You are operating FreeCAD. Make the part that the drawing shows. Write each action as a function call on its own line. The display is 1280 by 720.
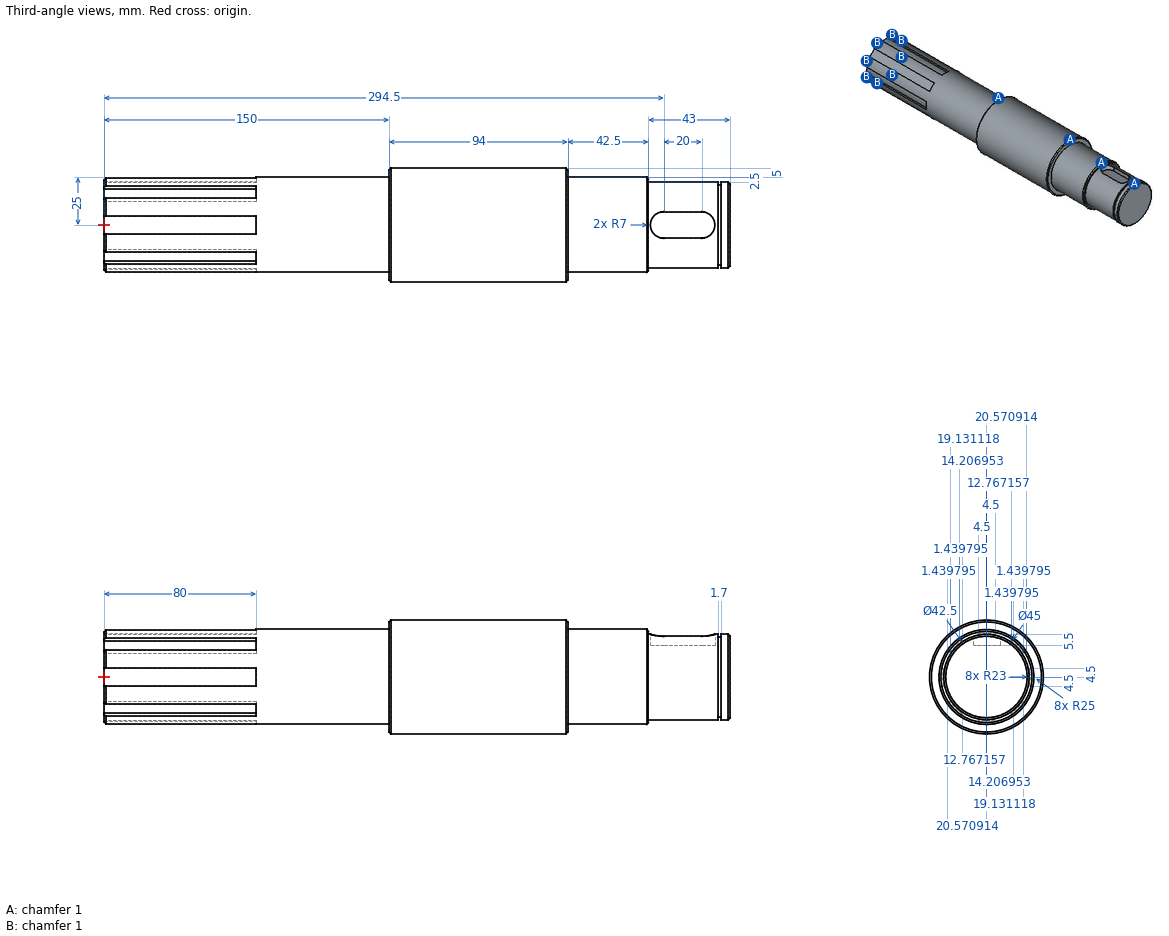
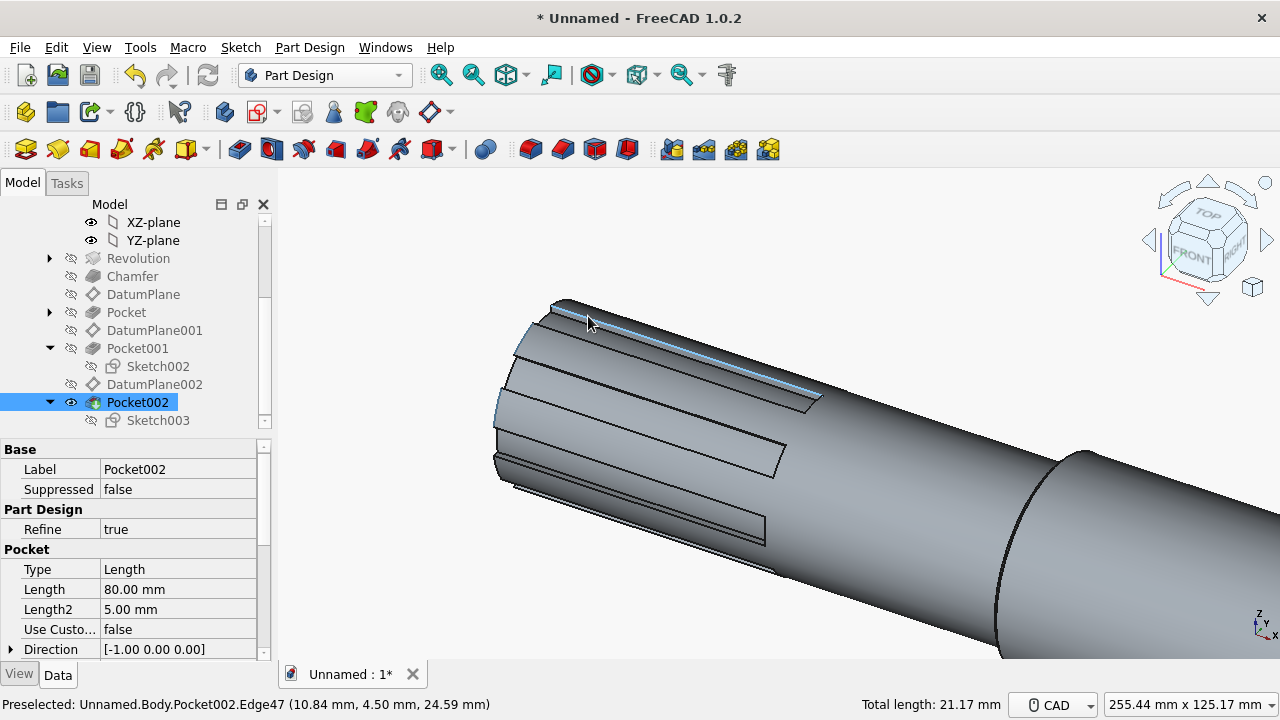
click(499, 475, ctrl)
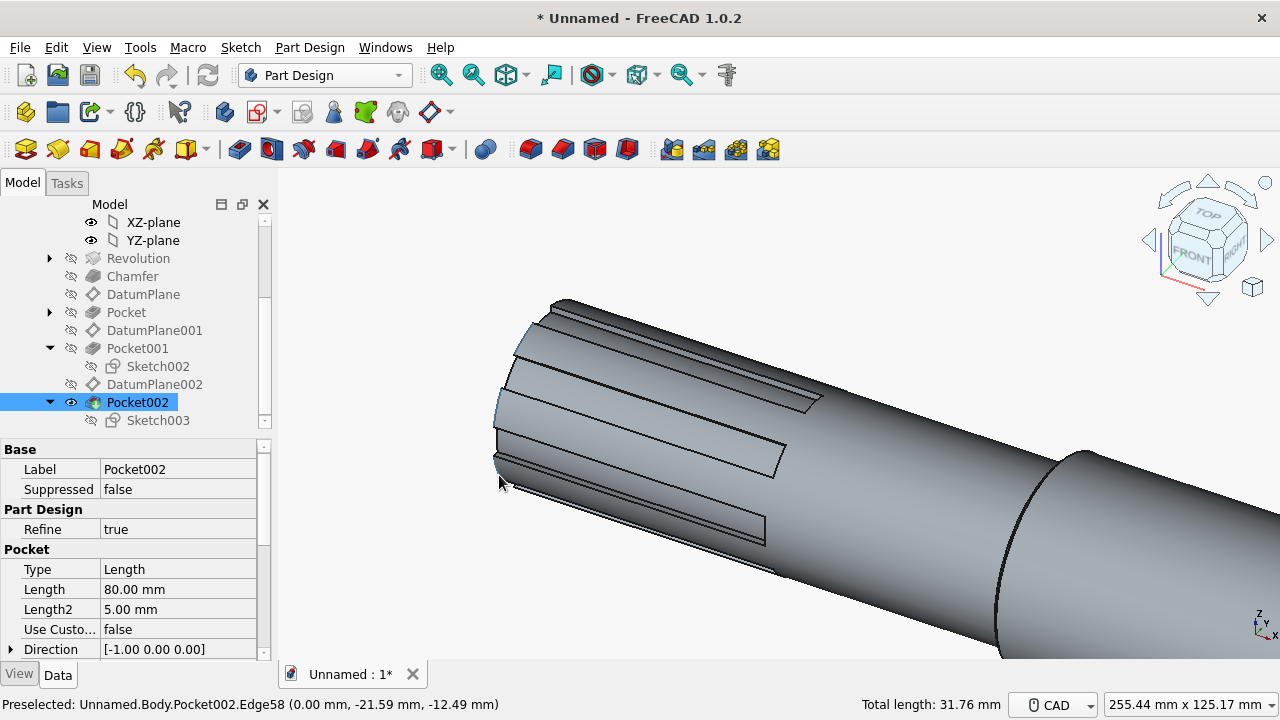
click(442, 76)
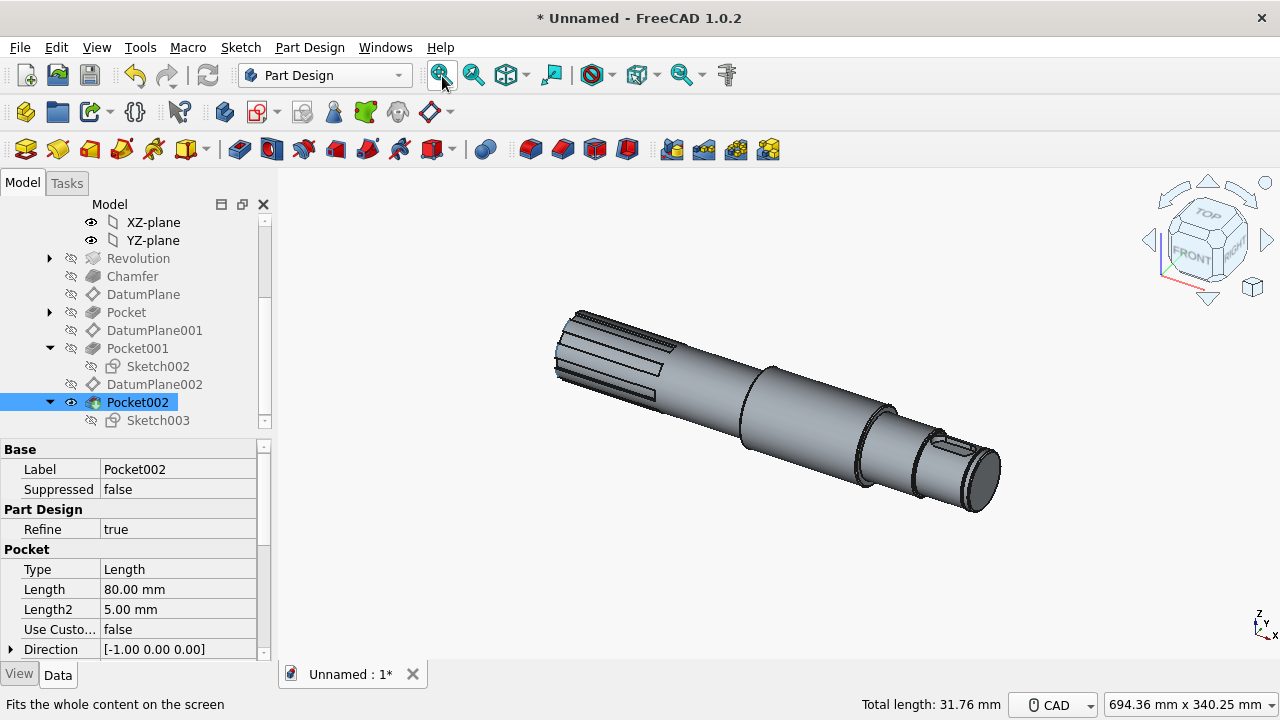
key(0)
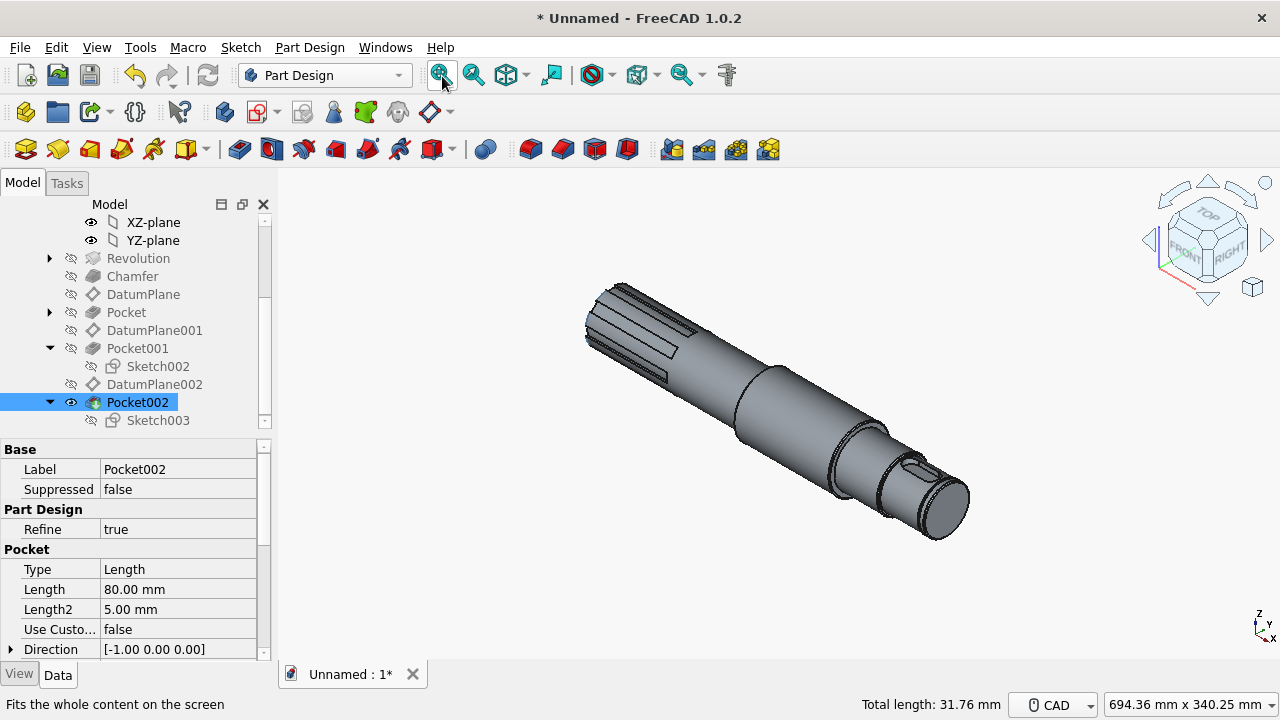
scroll(634, 291, up, 5)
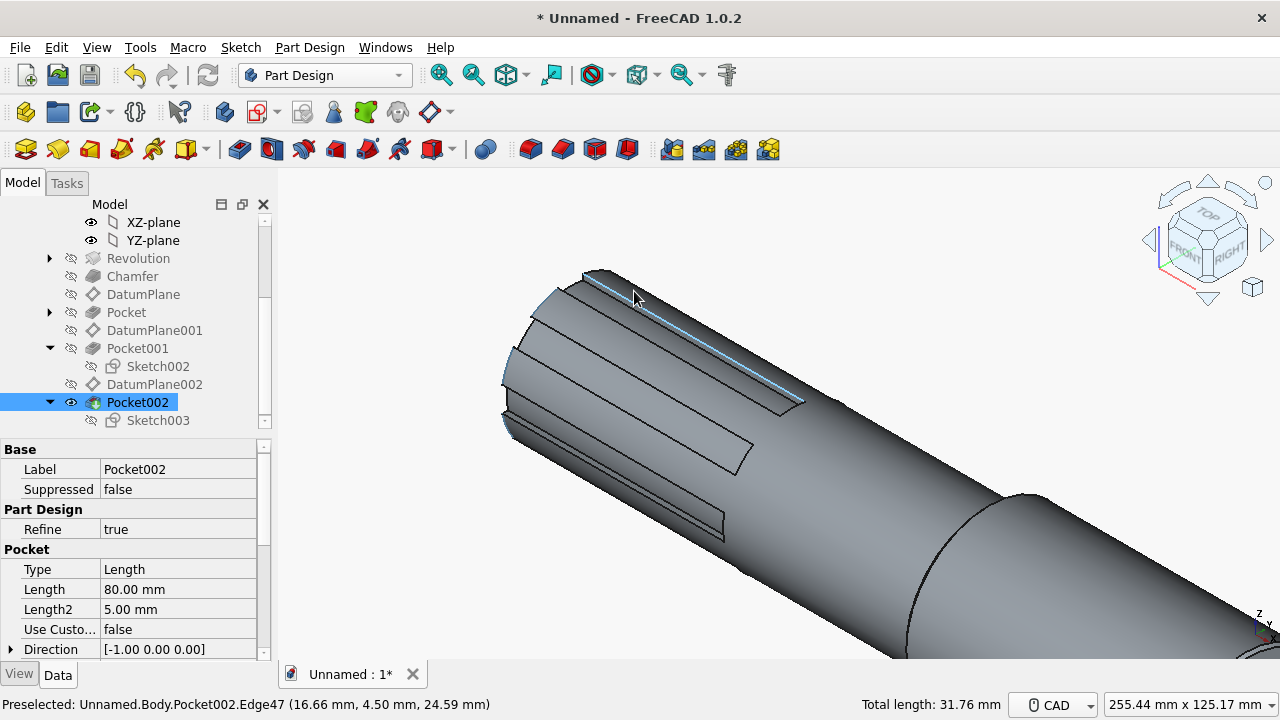
click(442, 76)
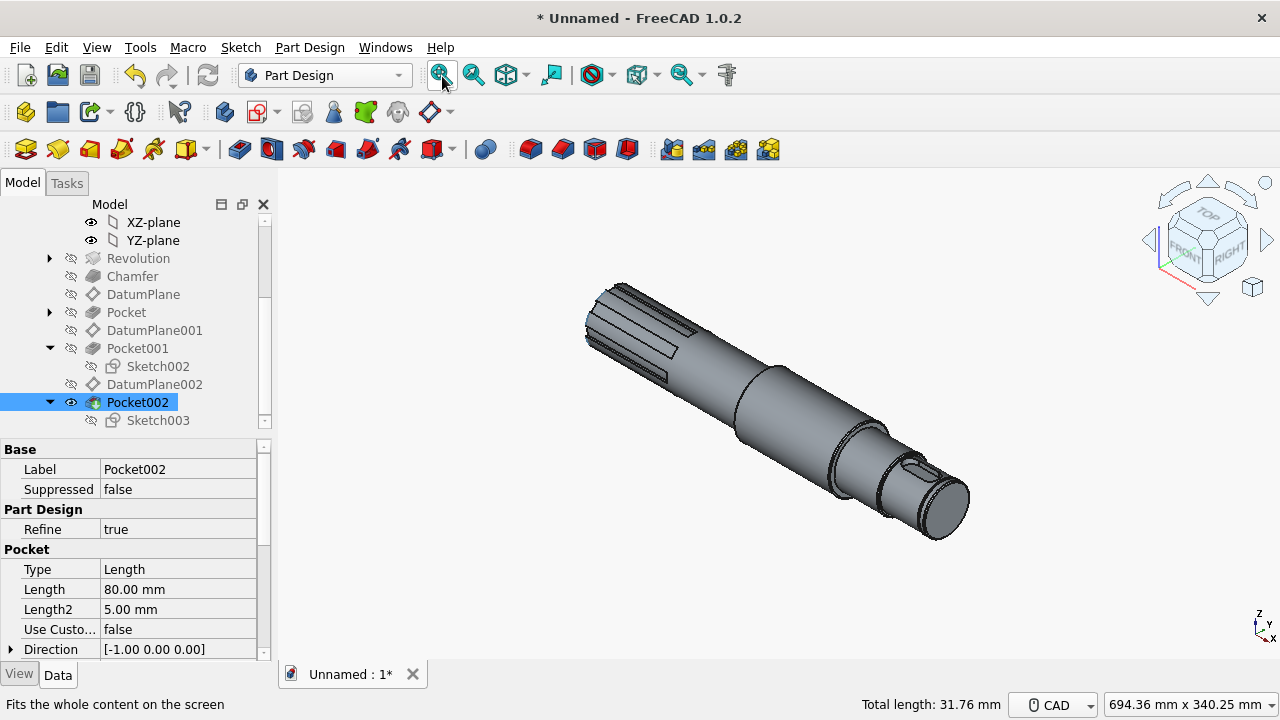
key(2)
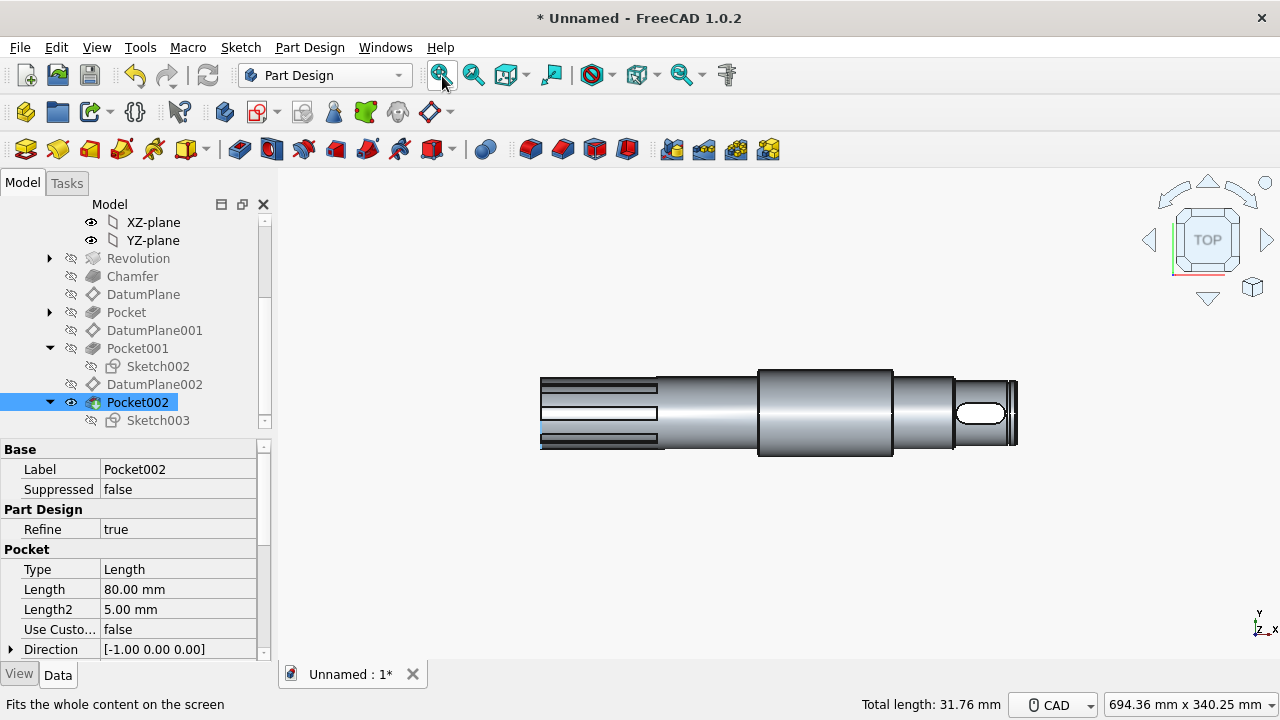
click(541, 399, ctrl)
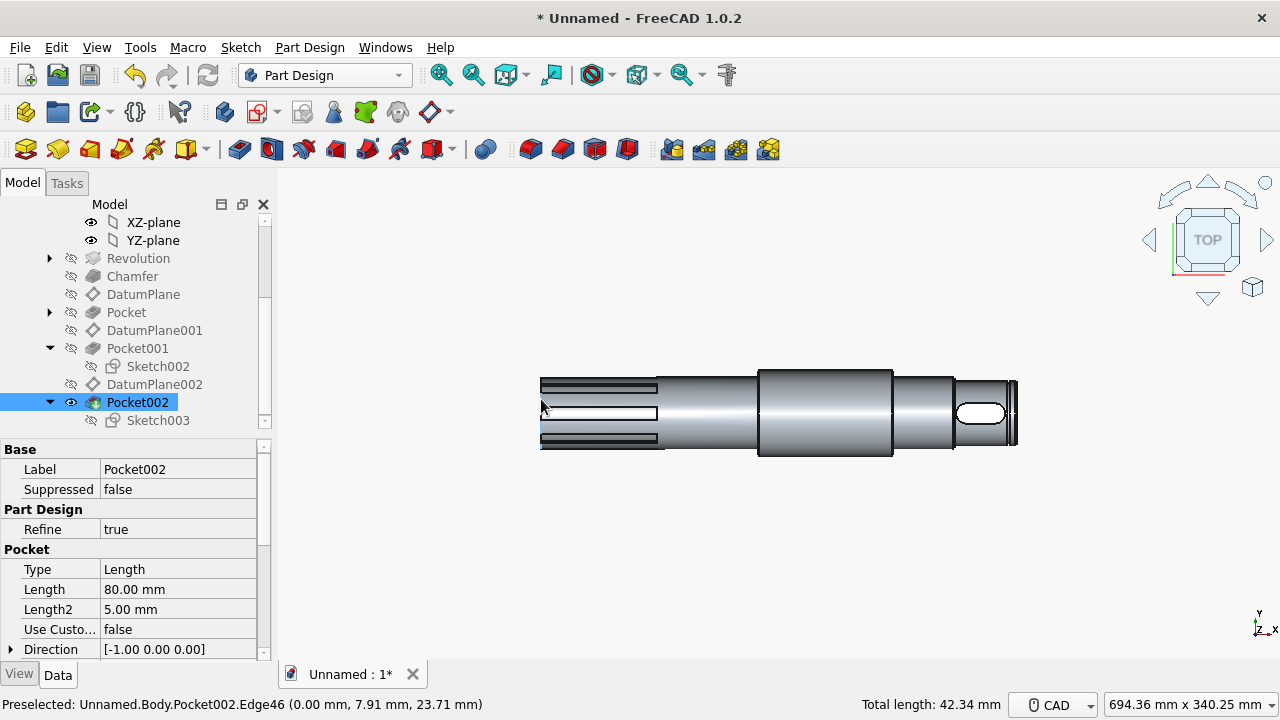
scroll(541, 379, up, 5)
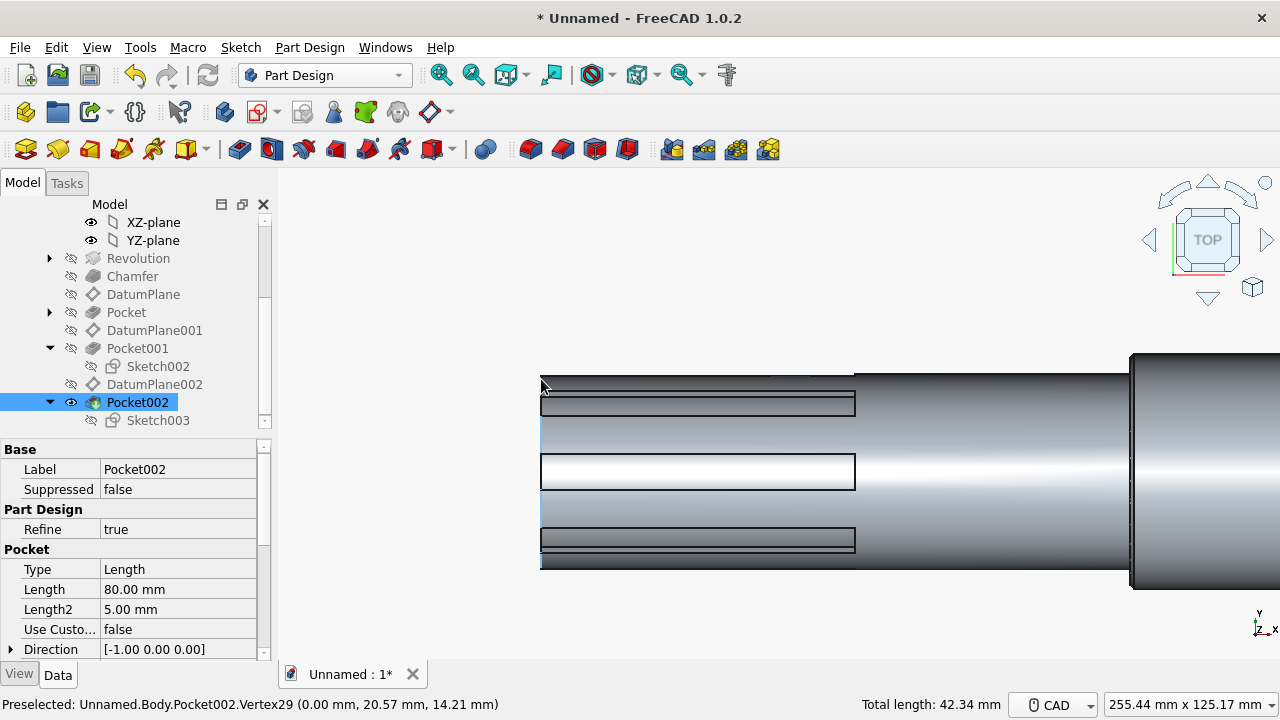
click(541, 382, ctrl)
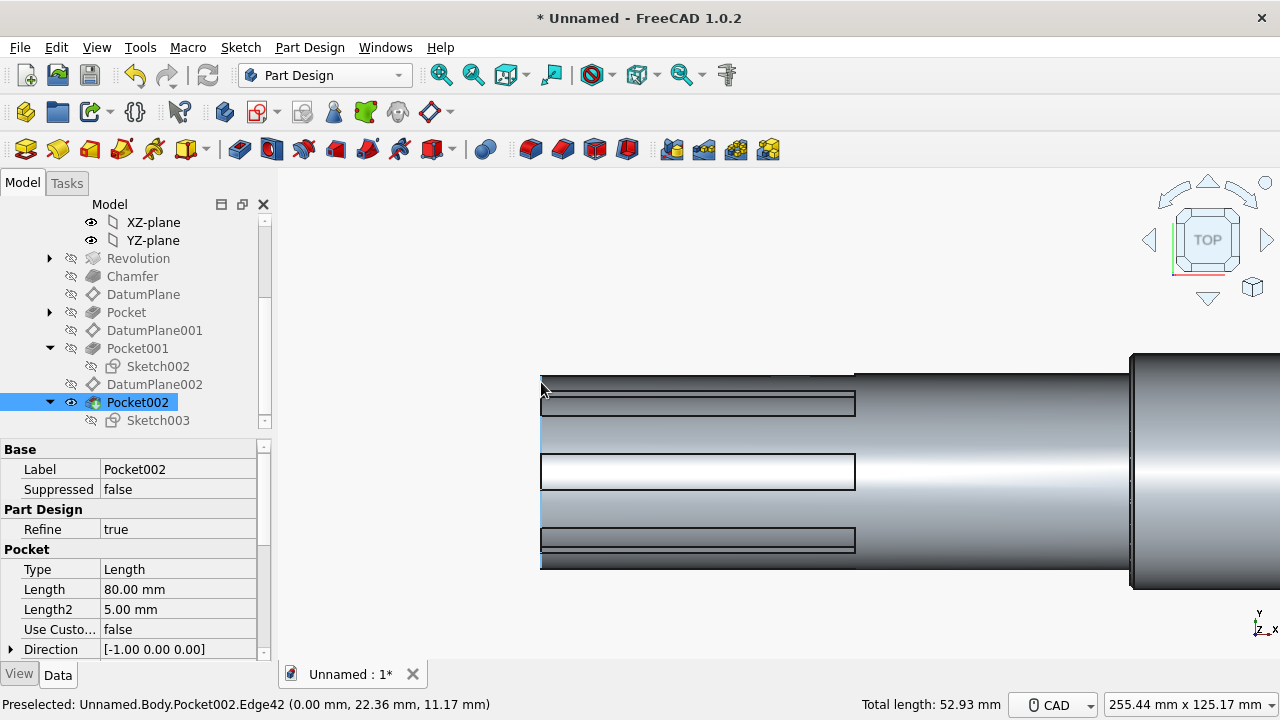
click(442, 76)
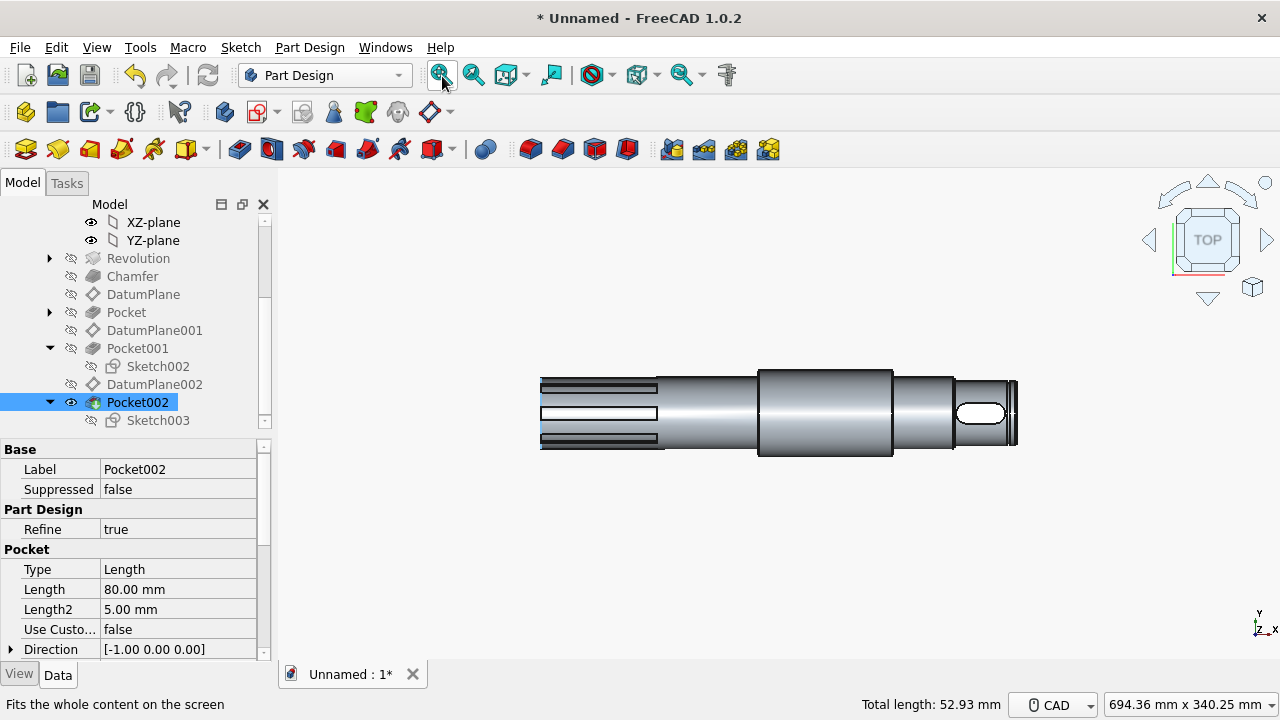
key(1)